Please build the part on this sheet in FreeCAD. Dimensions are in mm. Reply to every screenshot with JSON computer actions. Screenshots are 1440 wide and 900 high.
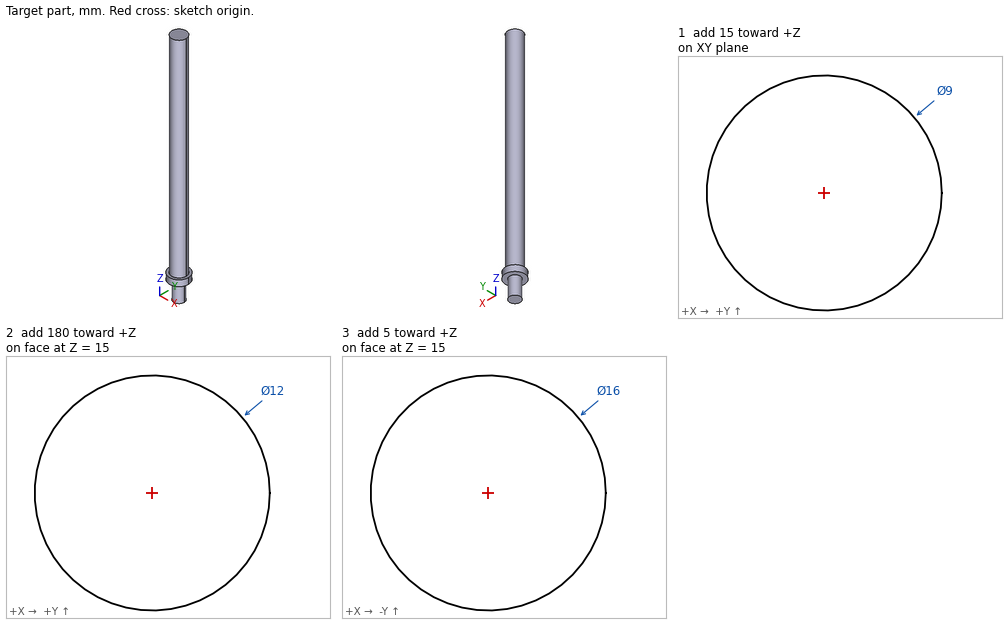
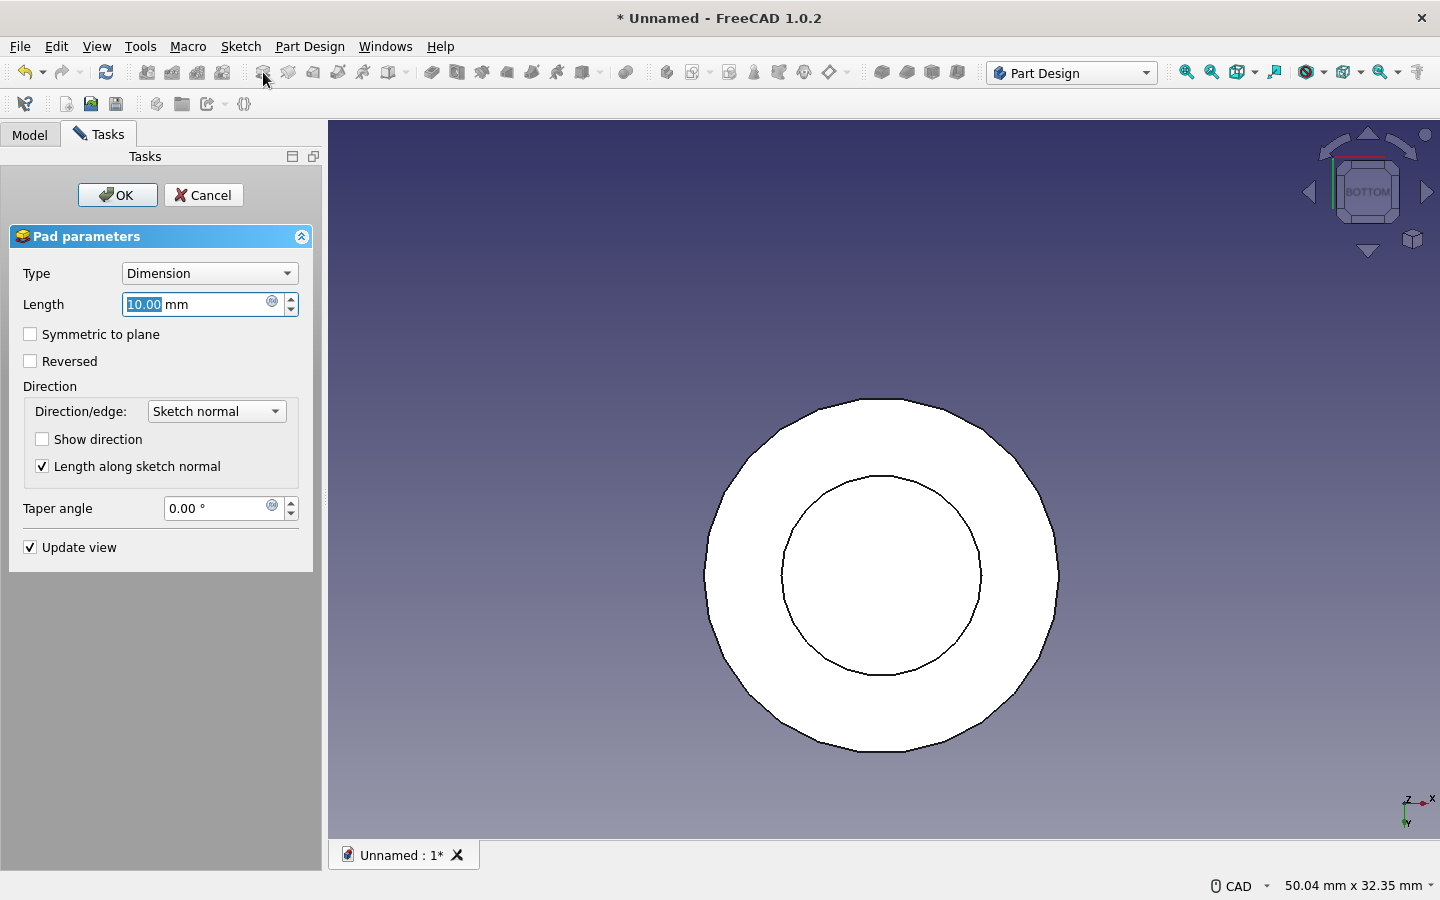
{"action": "type", "text": "5"}
{"action": "key", "text": "Tab"}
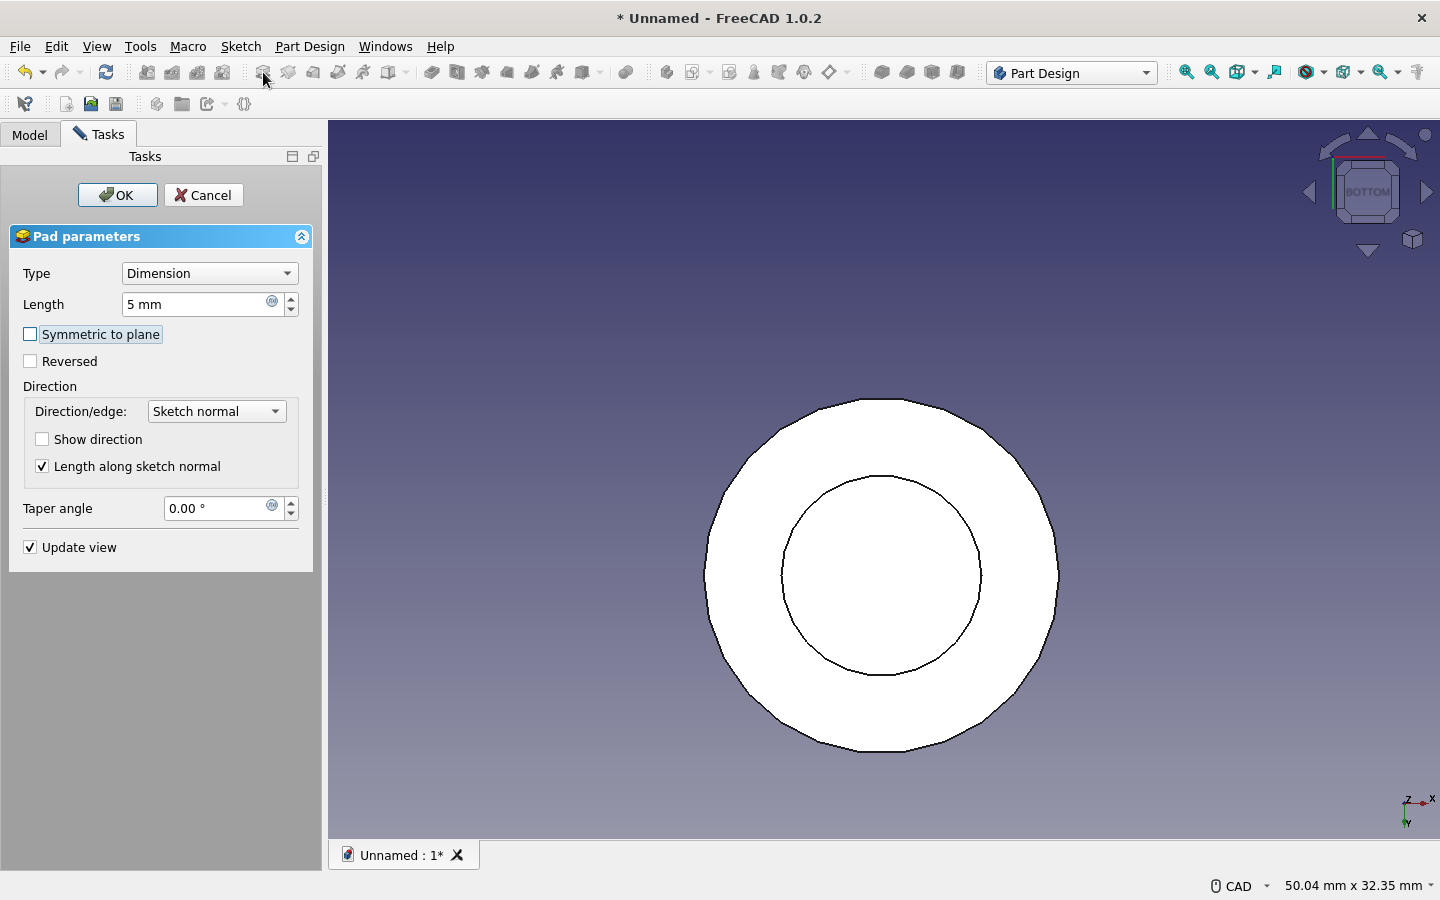
{"action": "left_click", "coordinate": [31, 361]}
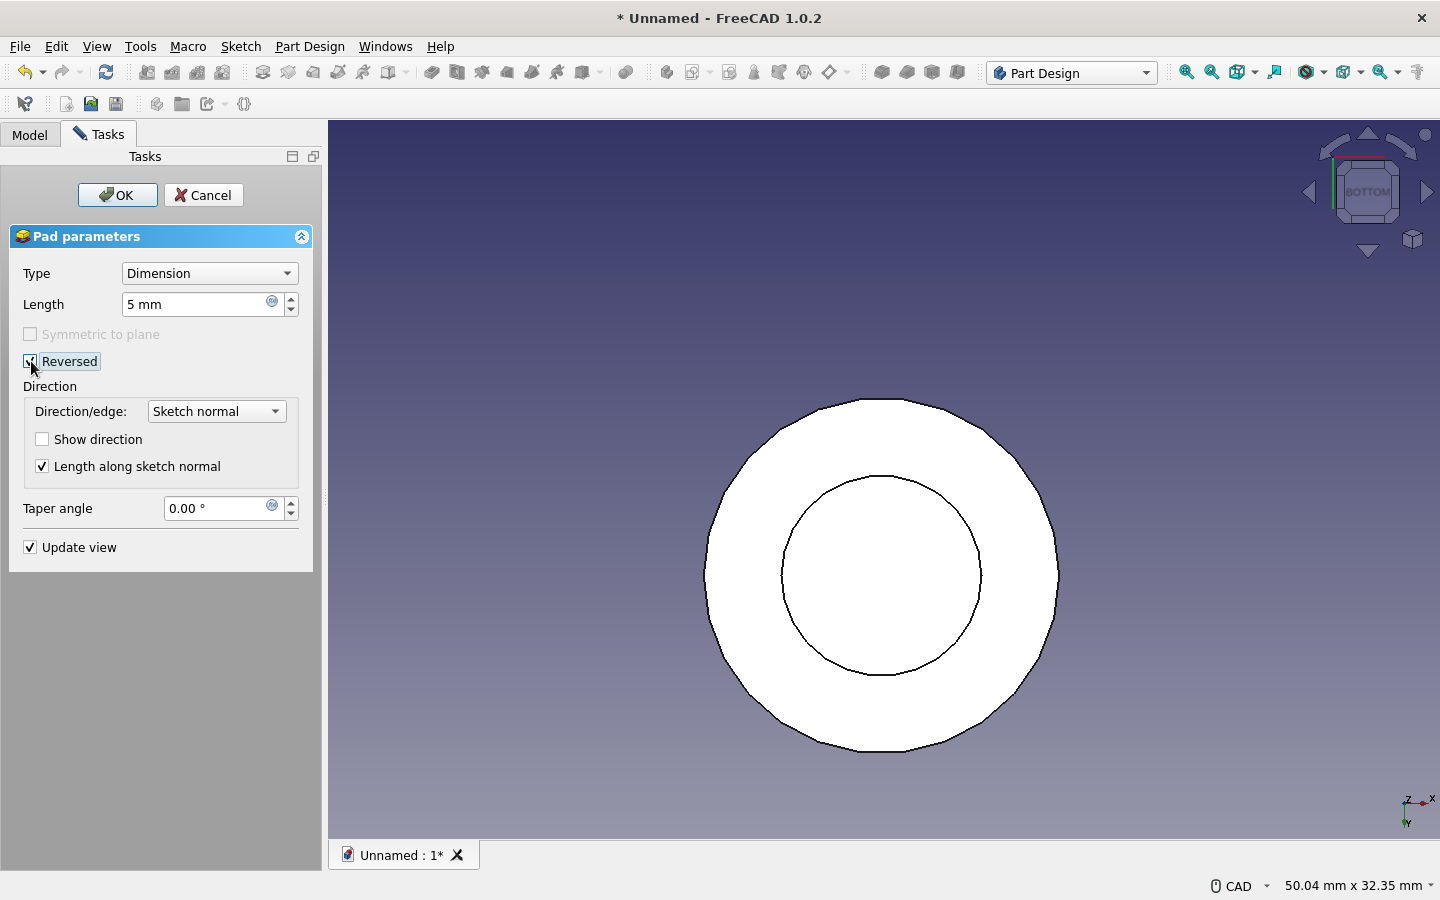
{"action": "left_click", "coordinate": [118, 195]}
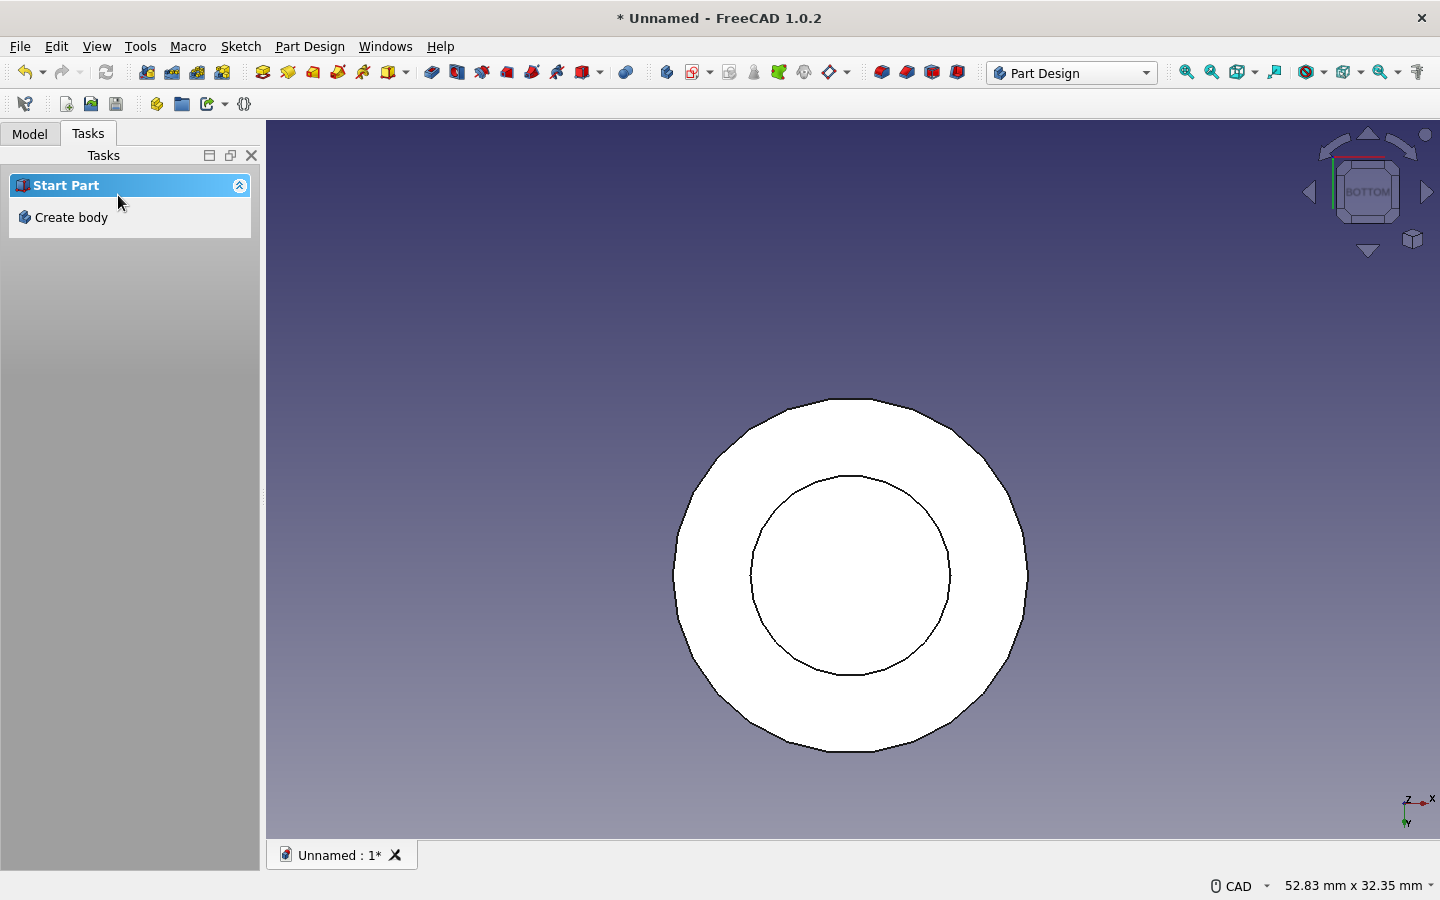
{"action": "key", "text": "0"}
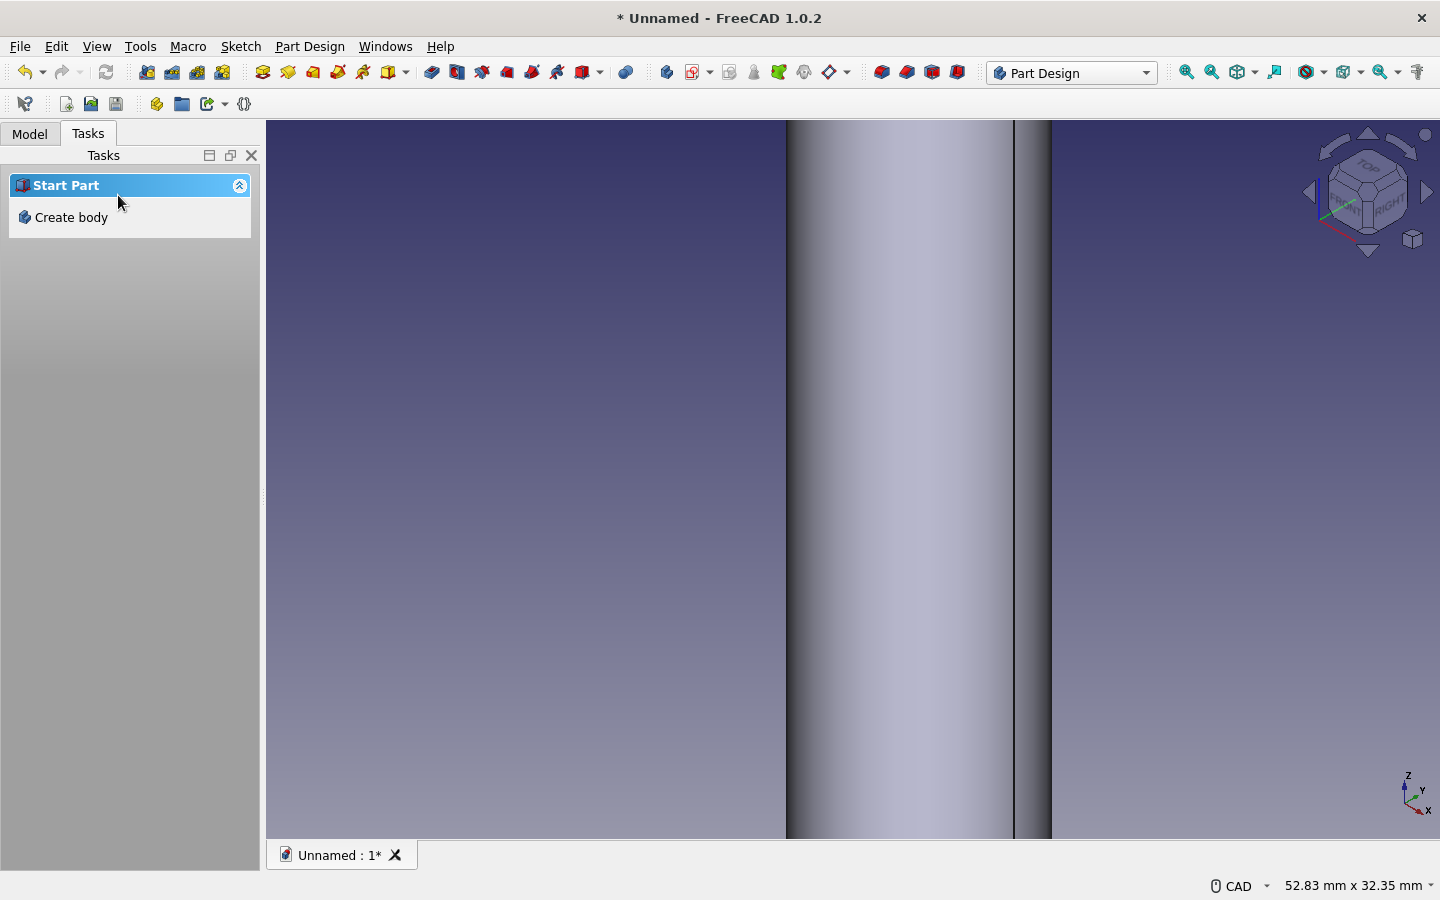
{"action": "key", "text": "v f"}